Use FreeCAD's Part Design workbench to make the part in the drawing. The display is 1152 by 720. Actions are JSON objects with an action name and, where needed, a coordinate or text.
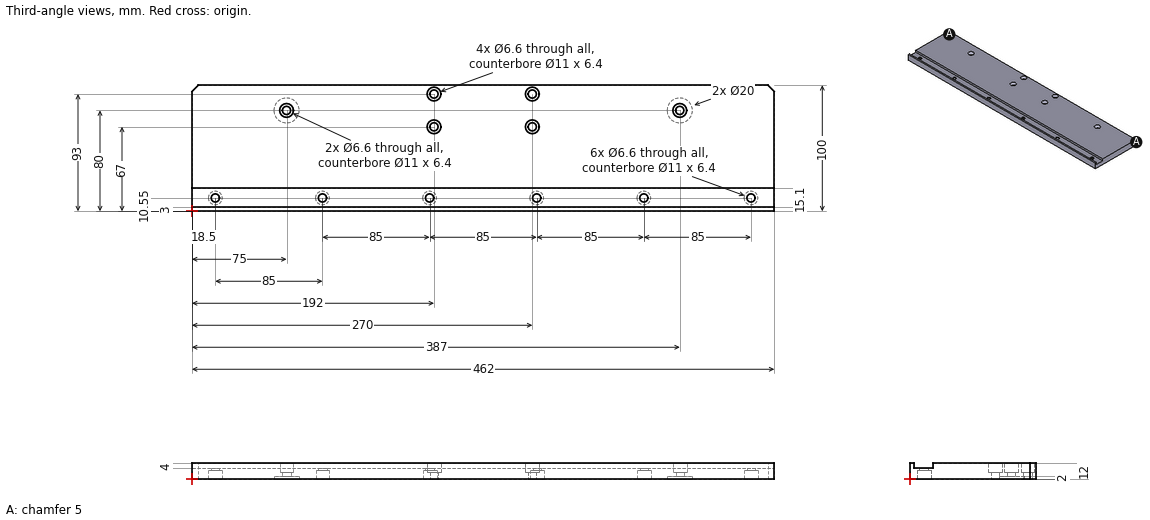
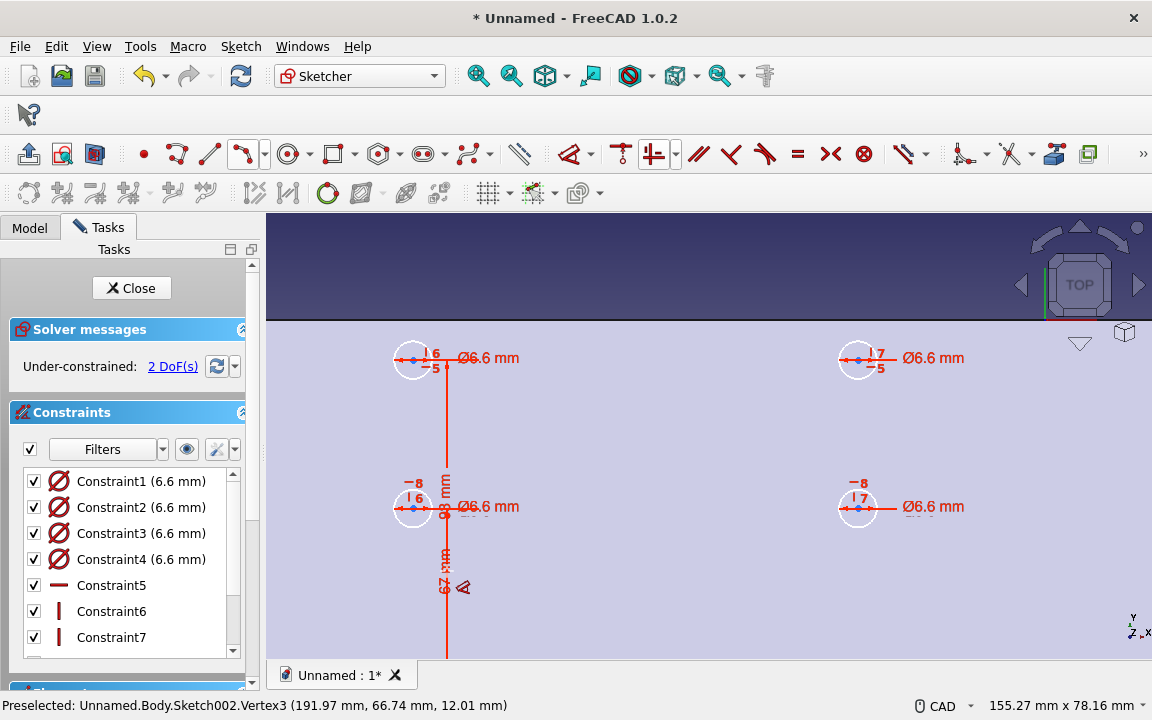
{"action": "left_click", "coordinate": [413, 360]}
{"action": "left_click", "coordinate": [354, 326]}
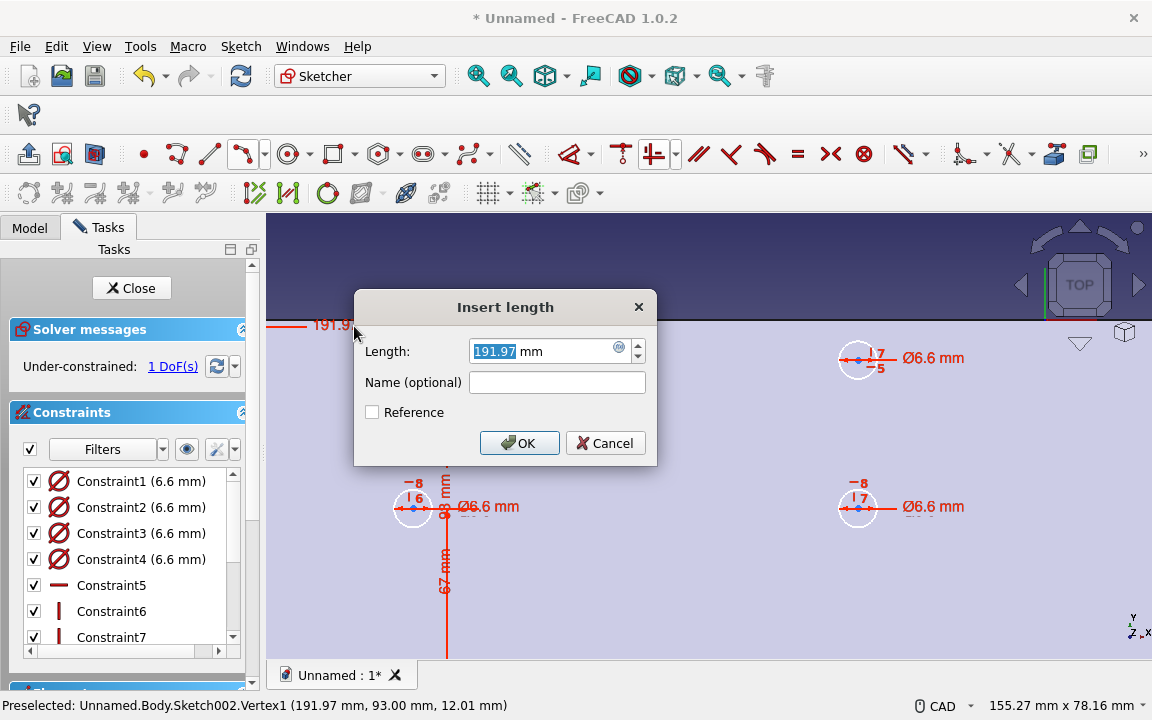
{"action": "type", "text": "192"}
{"action": "key", "text": "Return"}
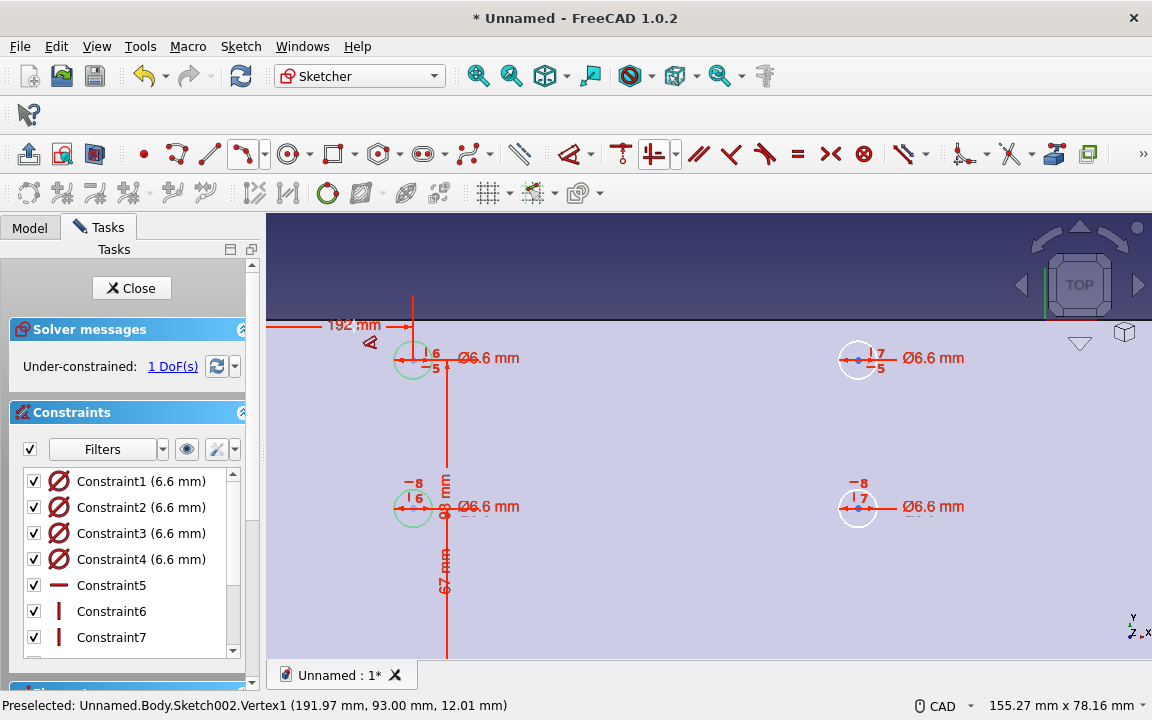
{"action": "left_click", "coordinate": [858, 360]}
{"action": "left_click", "coordinate": [576, 326]}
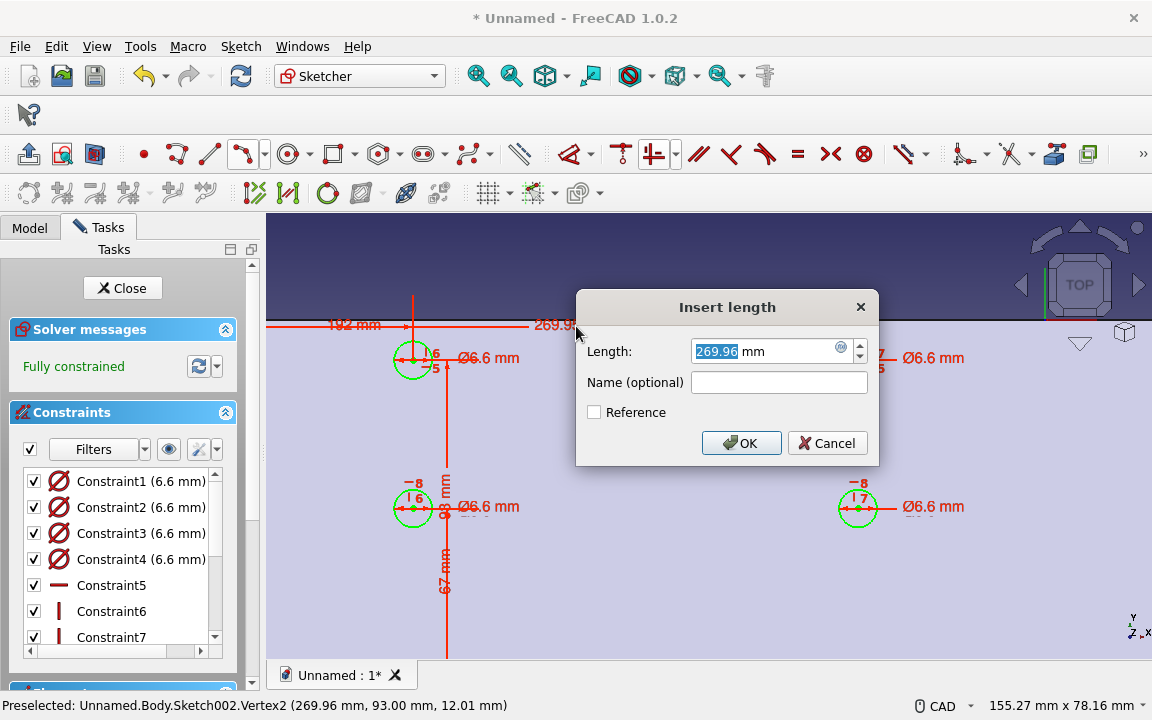
{"action": "type", "text": "270"}
{"action": "key", "text": "Return"}
{"action": "key", "text": "Escape"}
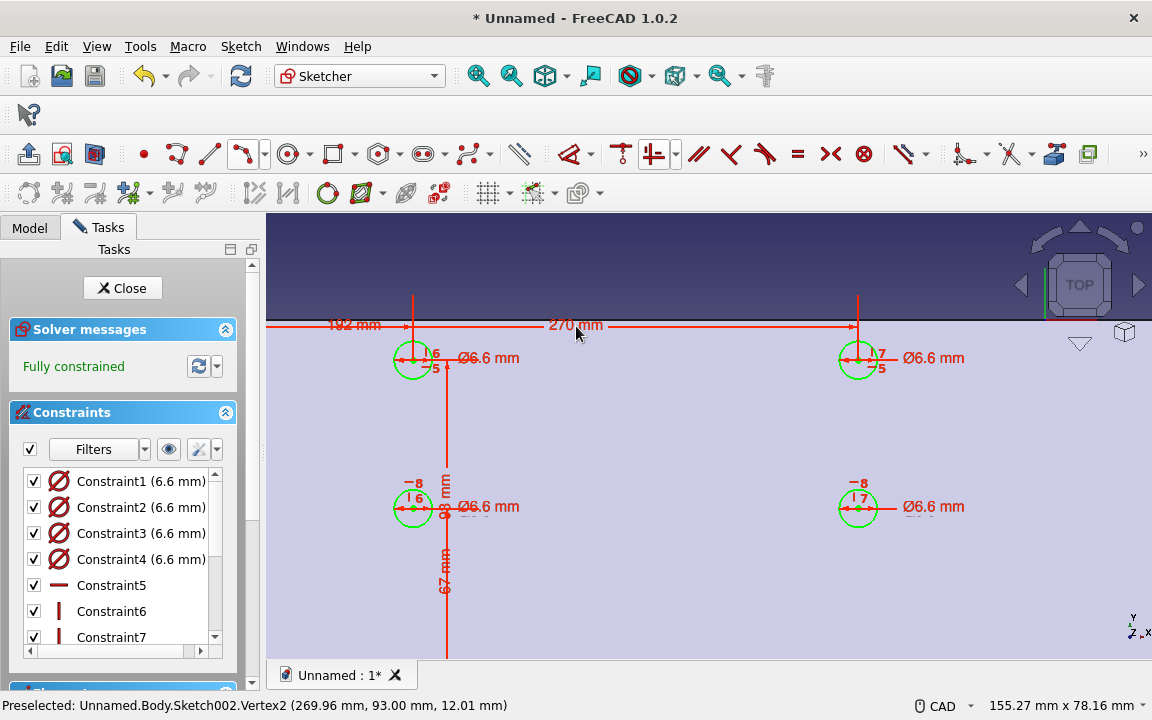
{"action": "left_click", "coordinate": [123, 288]}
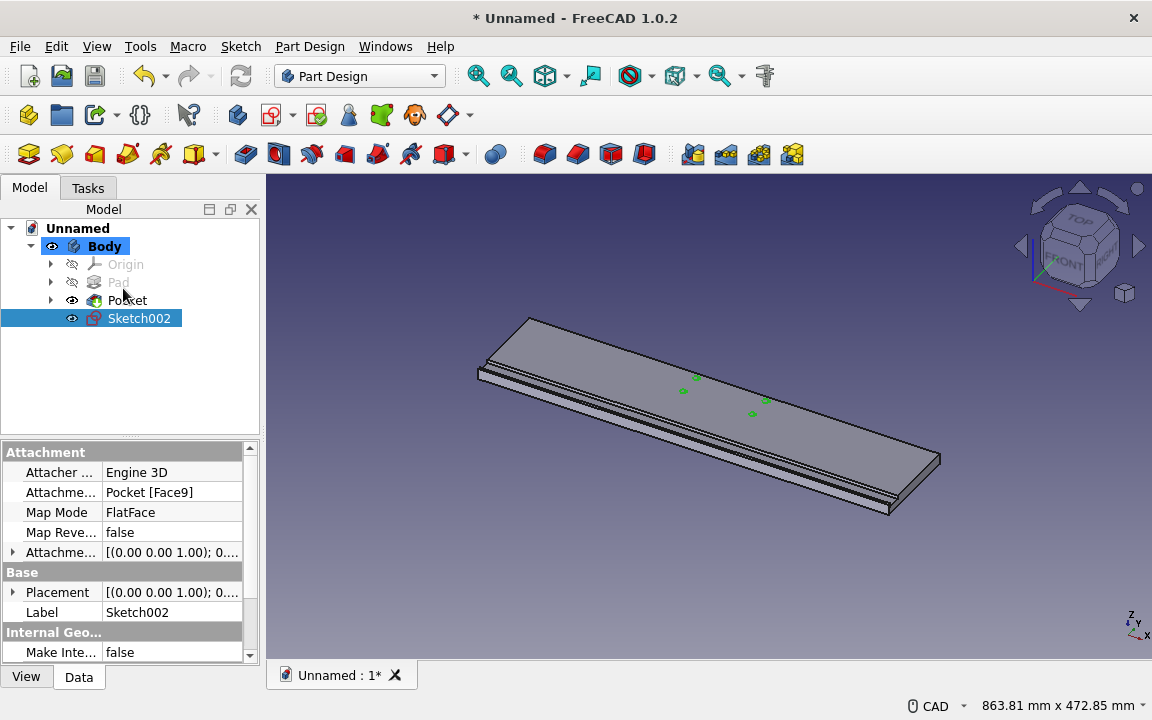
{"action": "left_click", "coordinate": [279, 154]}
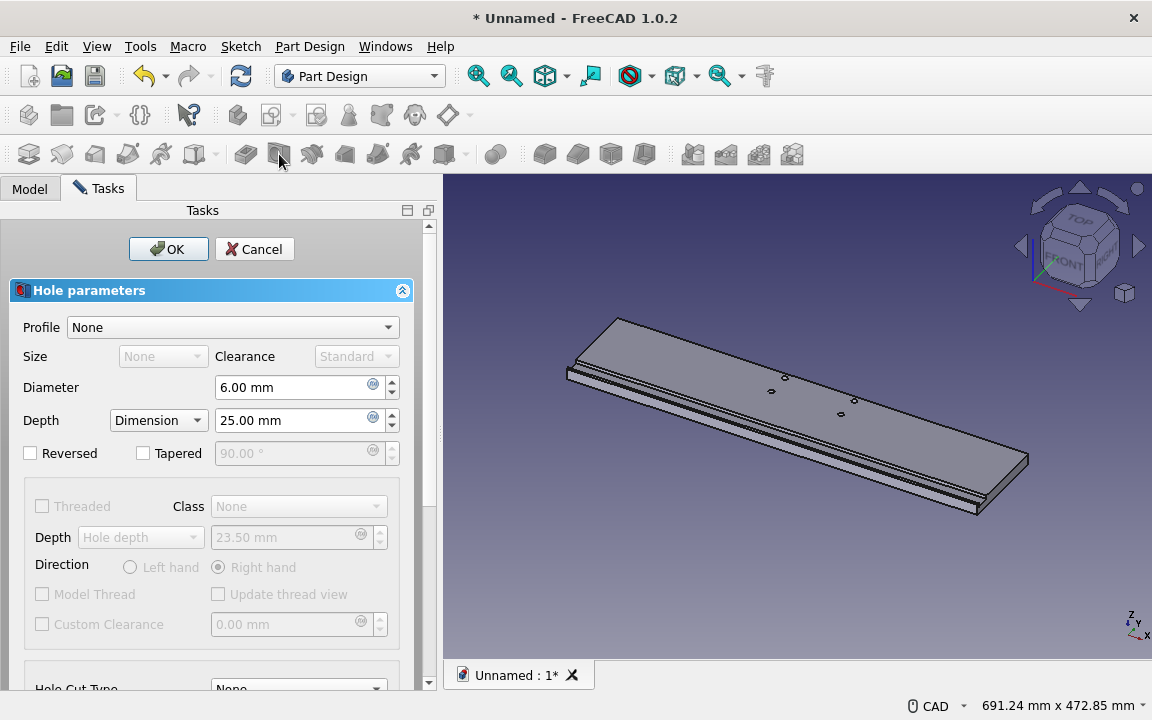
{"action": "triple_click", "coordinate": [300, 388]}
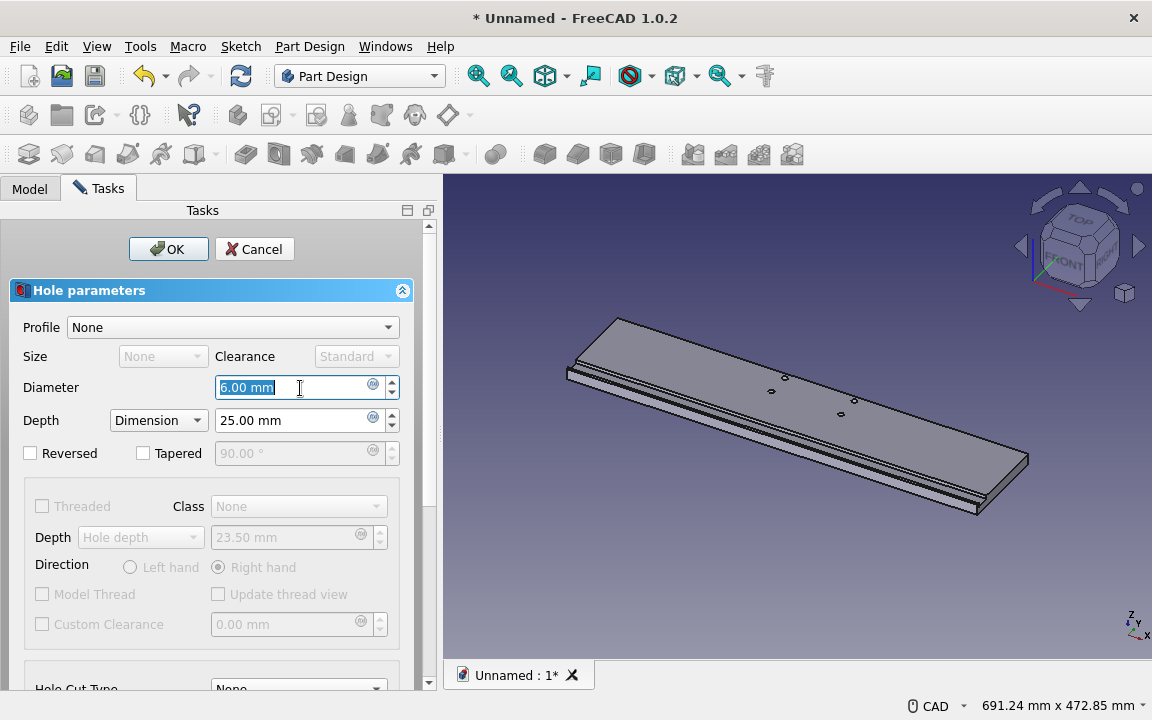
{"action": "type", "text": "6.6"}
{"action": "key", "text": "Tab"}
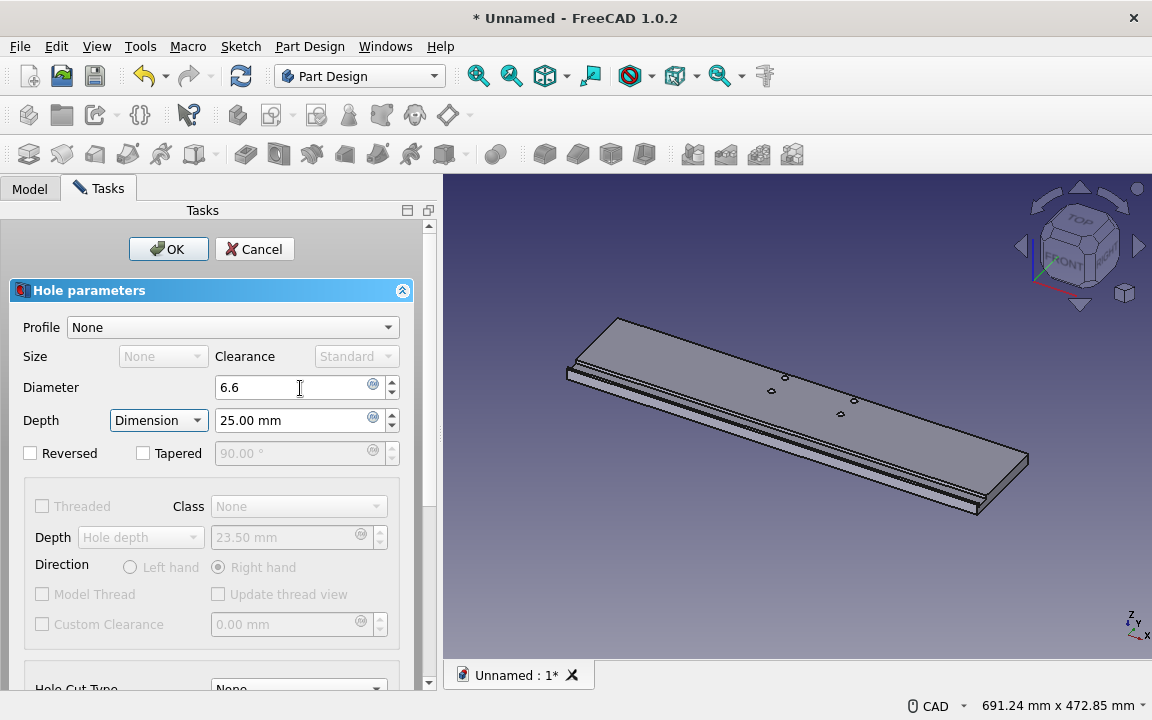
{"action": "left_click", "coordinate": [160, 420]}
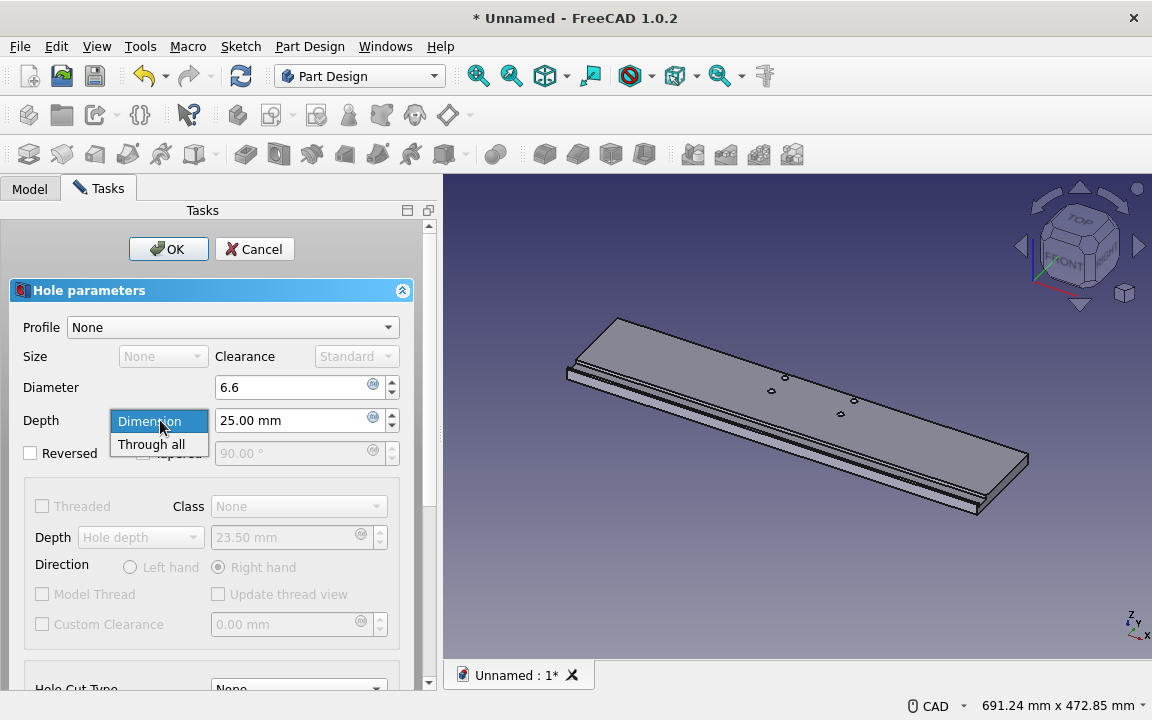
{"action": "left_click", "coordinate": [158, 444]}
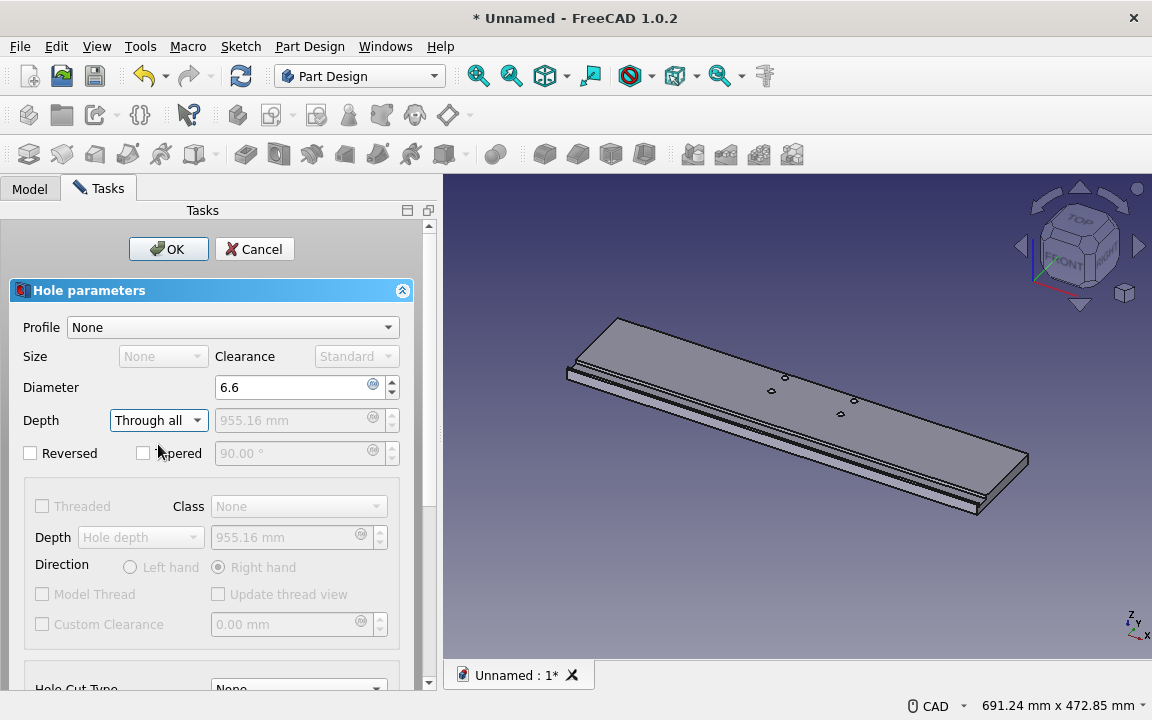
{"action": "scroll", "coordinate": [429, 455], "scroll_direction": "down", "scroll_amount": 2}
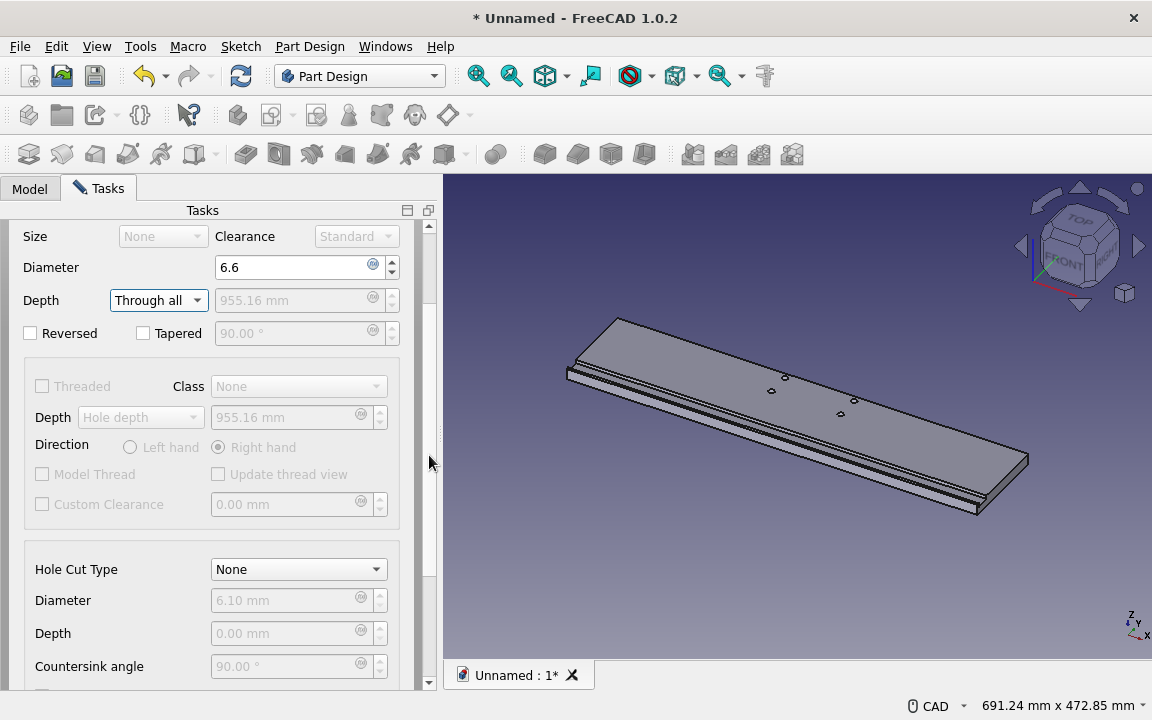
{"action": "left_click", "coordinate": [300, 570]}